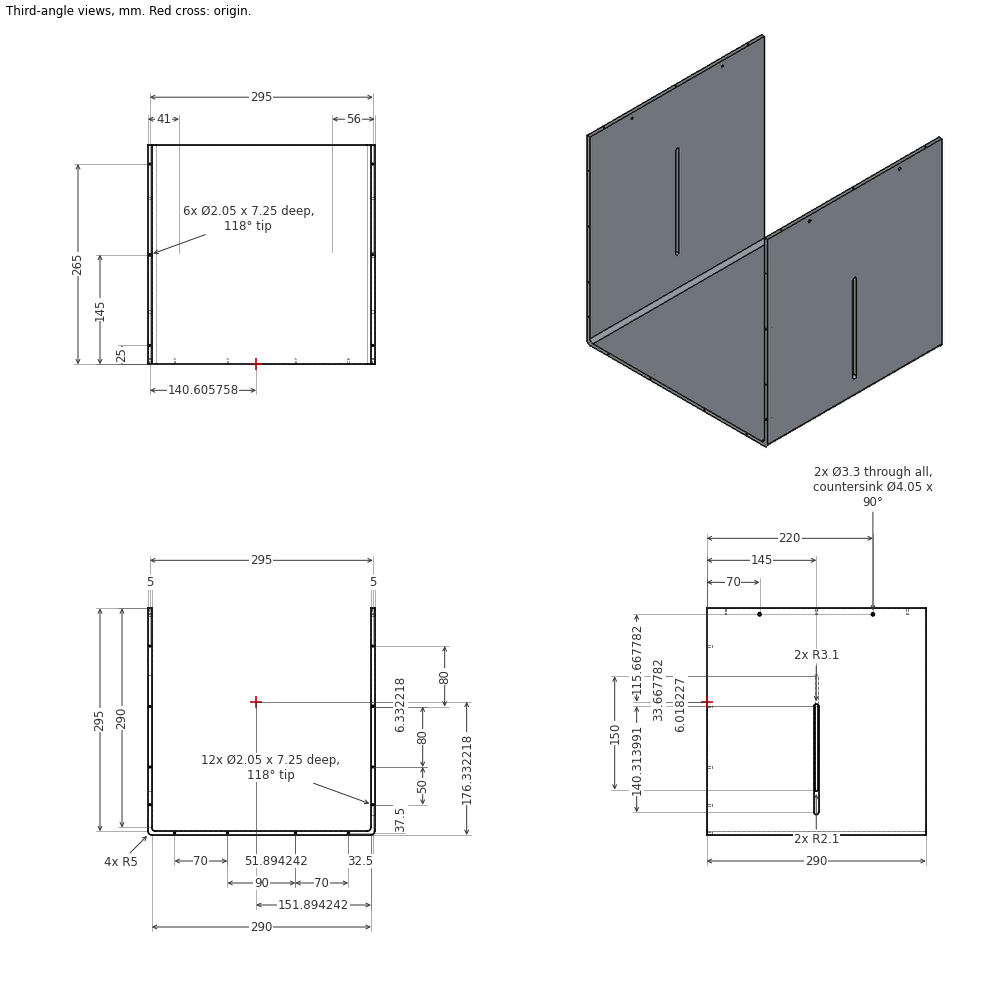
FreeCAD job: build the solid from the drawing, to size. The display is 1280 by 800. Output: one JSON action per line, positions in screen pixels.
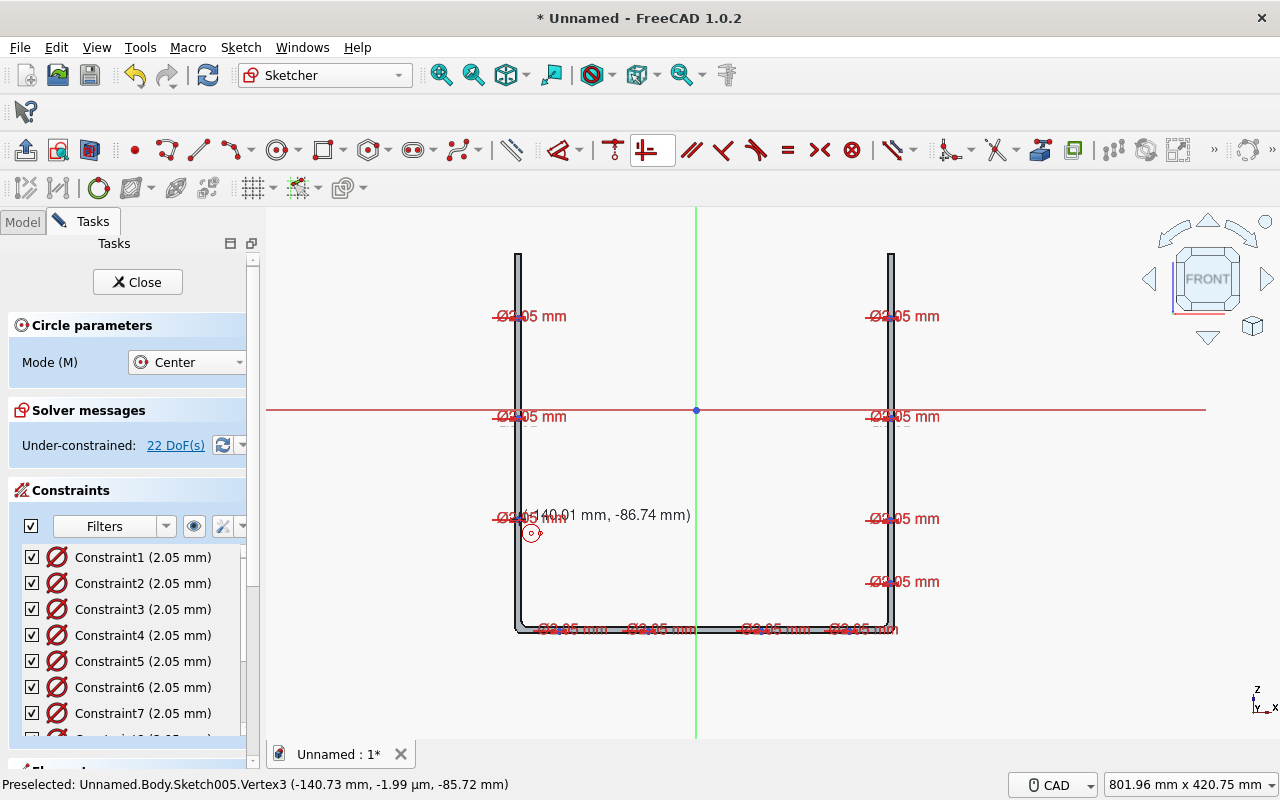
{"action": "scroll", "coordinate": [518, 583], "scroll_direction": "up", "scroll_amount": 15}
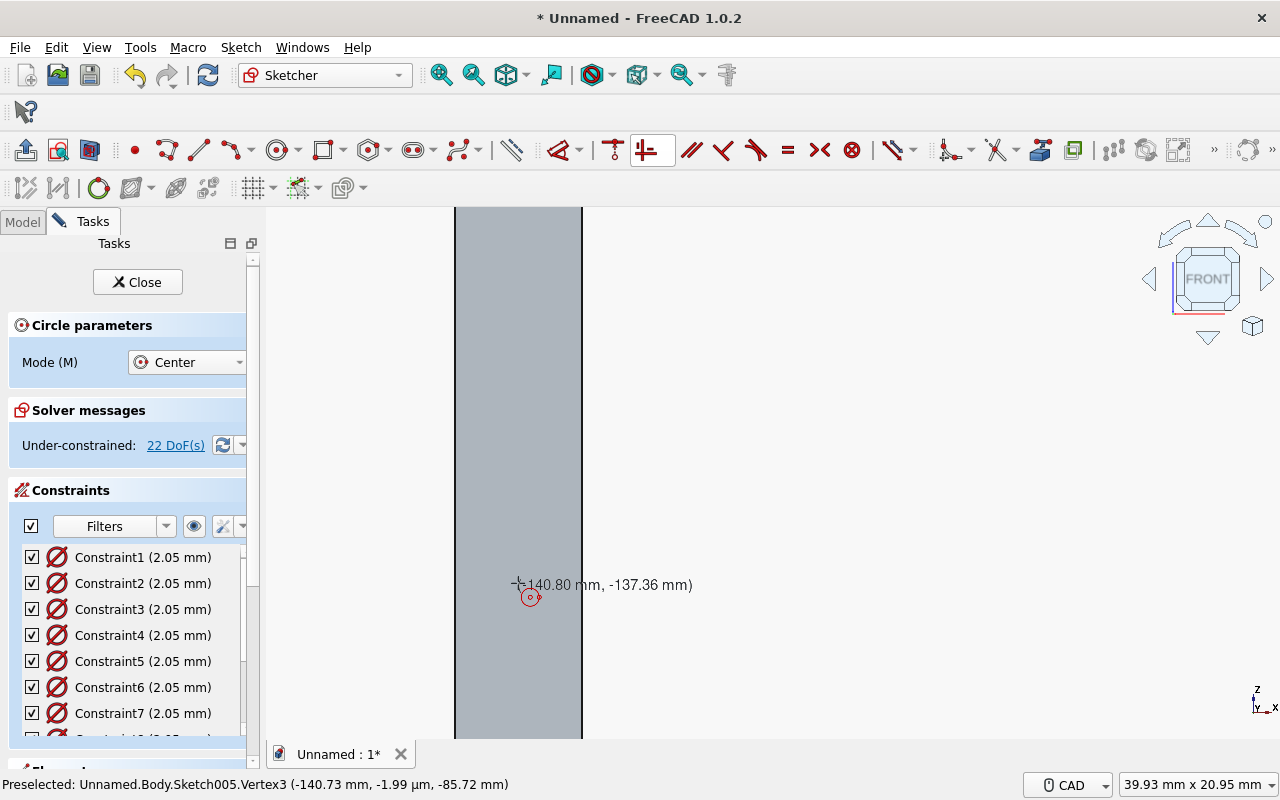
{"action": "scroll", "coordinate": [518, 583], "scroll_direction": "down", "scroll_amount": 15}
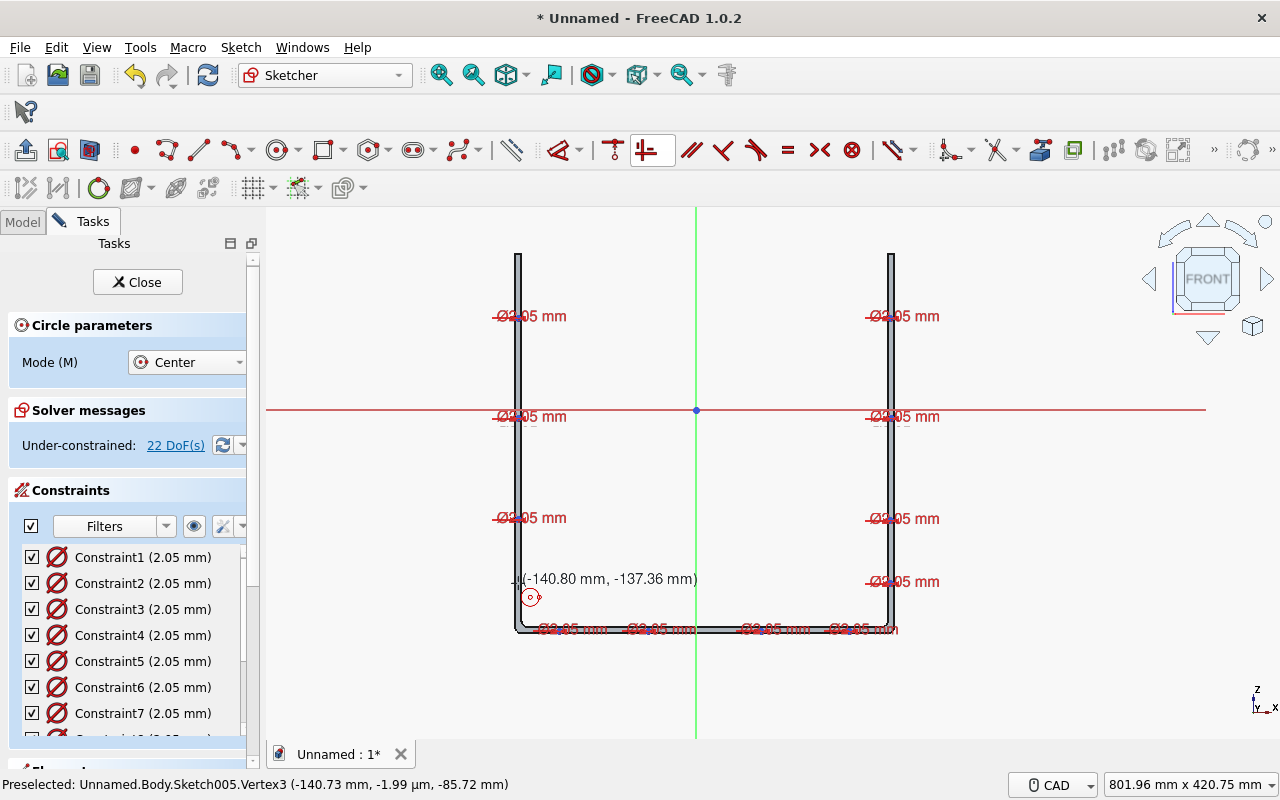
{"action": "left_click", "coordinate": [518, 583]}
{"action": "mouse_move", "coordinate": [519, 582]}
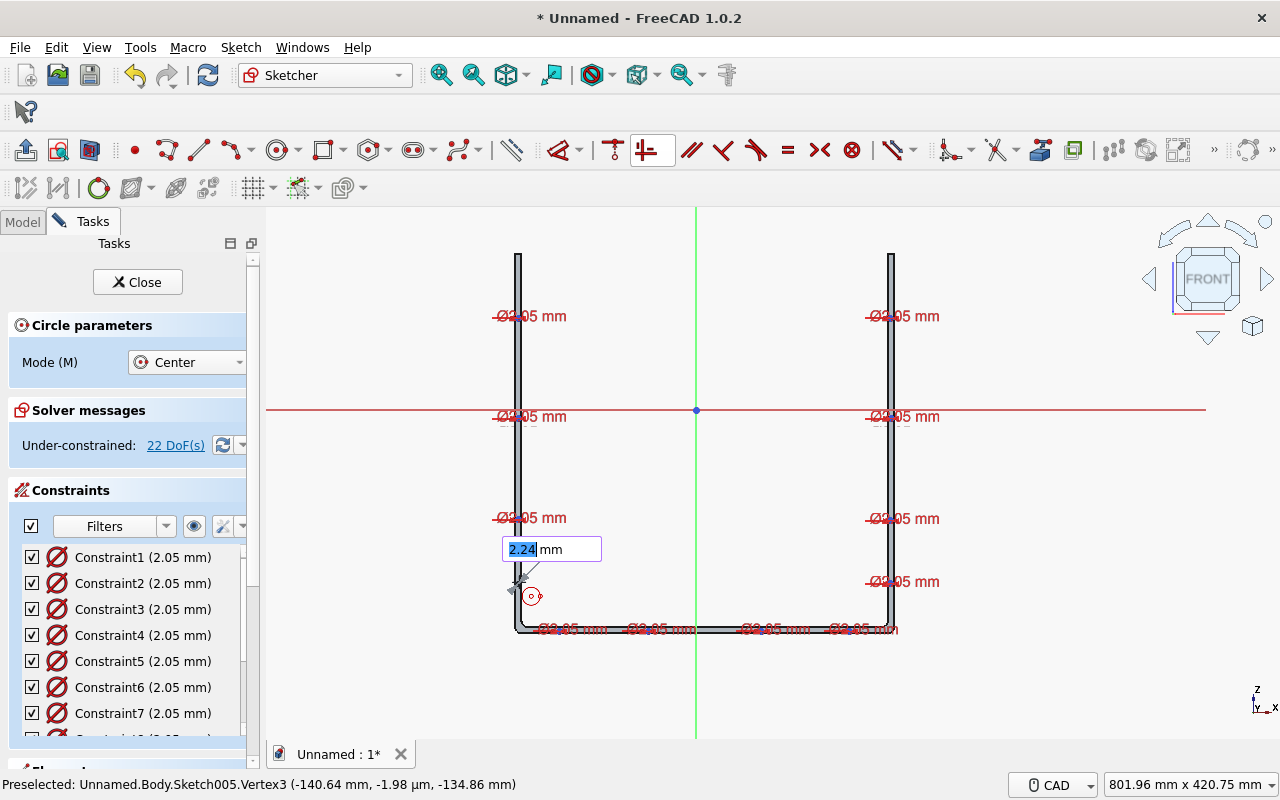
{"action": "type", "text": "2.05"}
{"action": "key", "text": "Return"}
{"action": "key", "text": "Escape"}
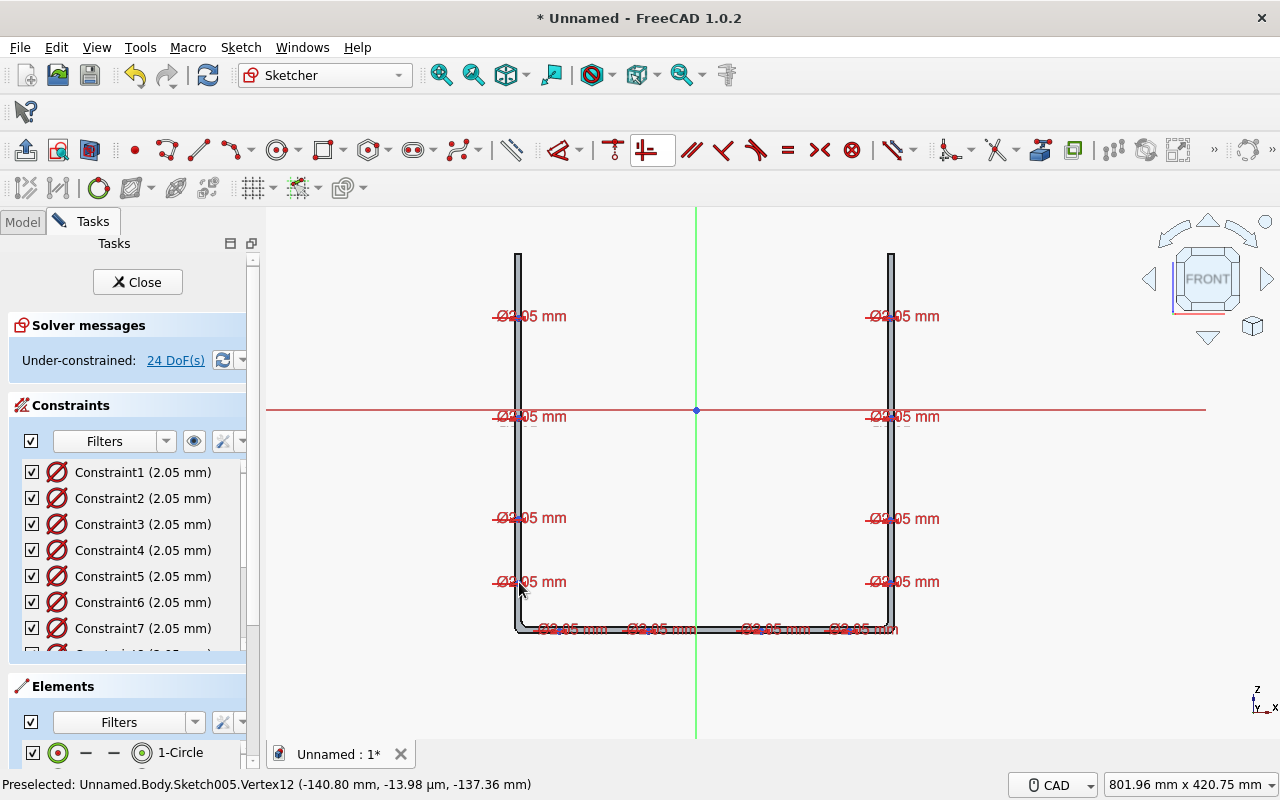
{"action": "left_click", "coordinate": [891, 584]}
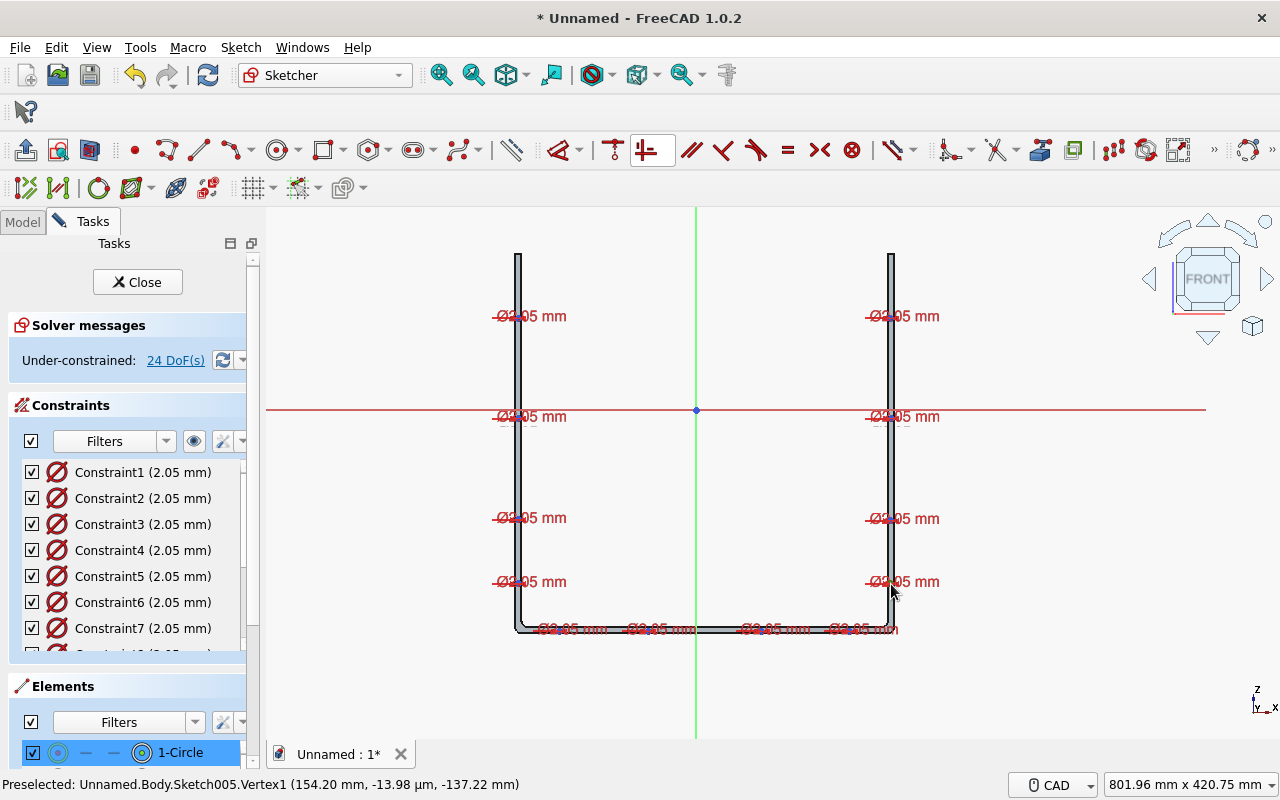
{"action": "left_click", "coordinate": [891, 521]}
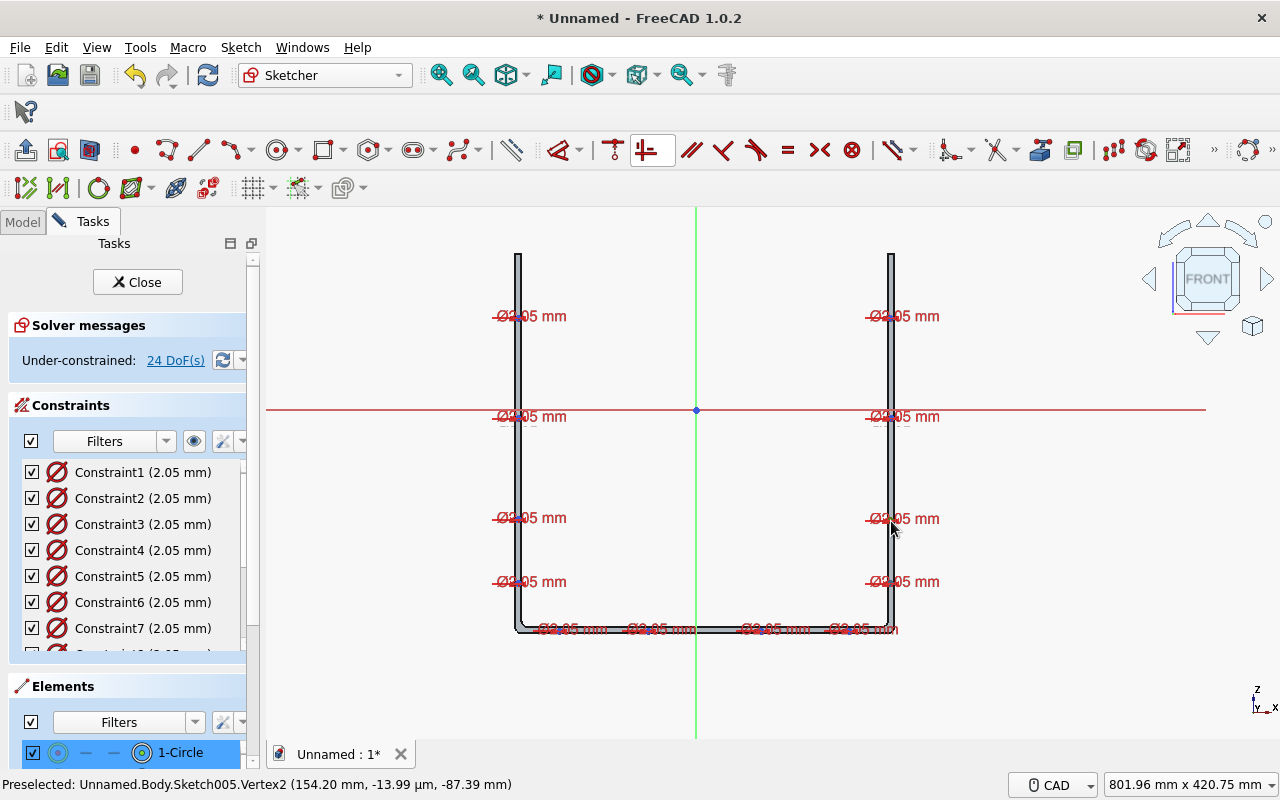
{"action": "left_click", "coordinate": [670, 150]}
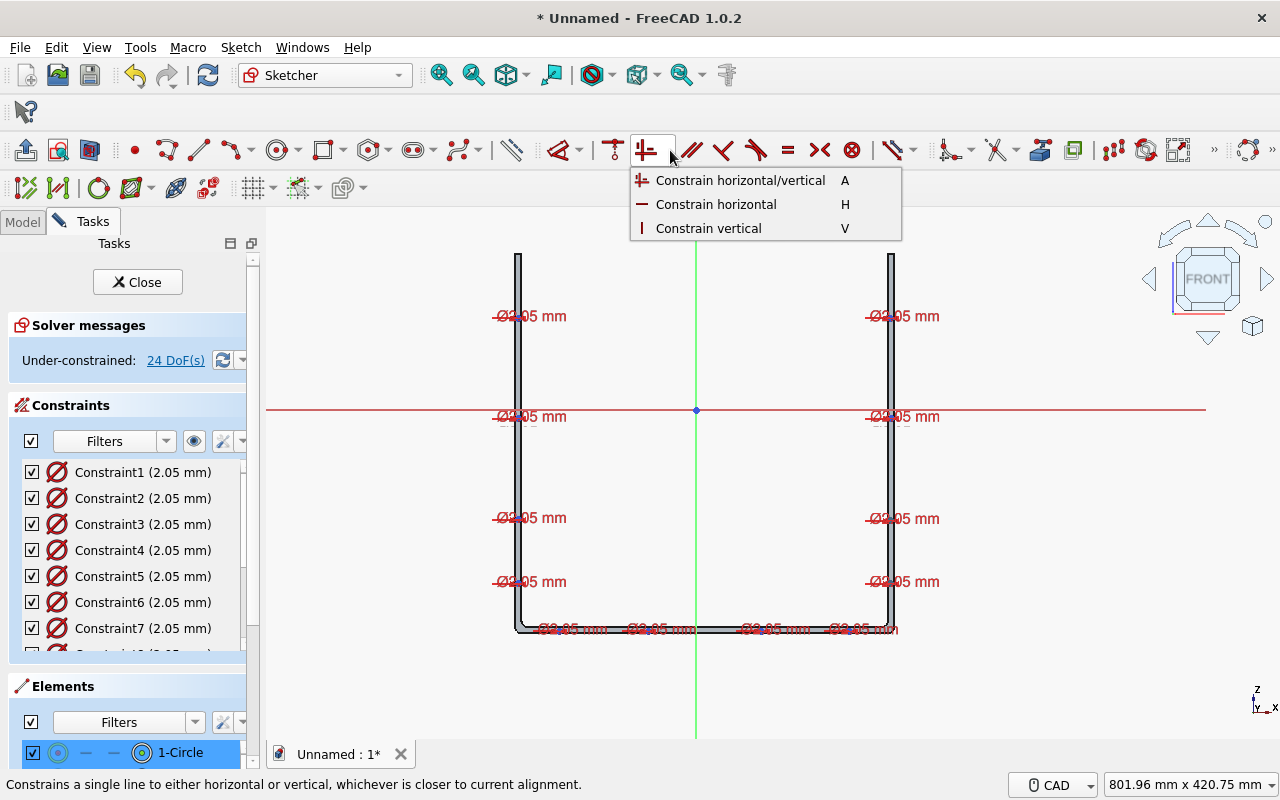
{"action": "left_click", "coordinate": [766, 228]}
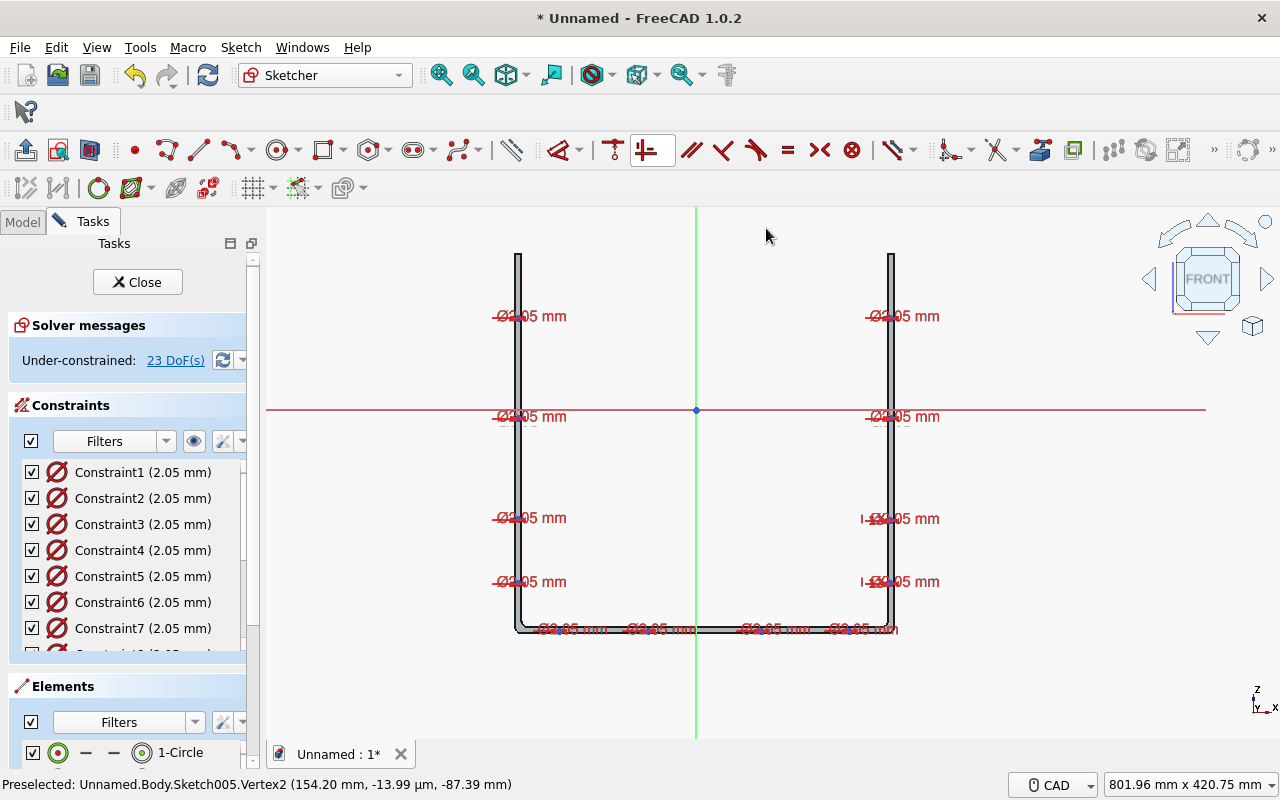
{"action": "left_click", "coordinate": [891, 521]}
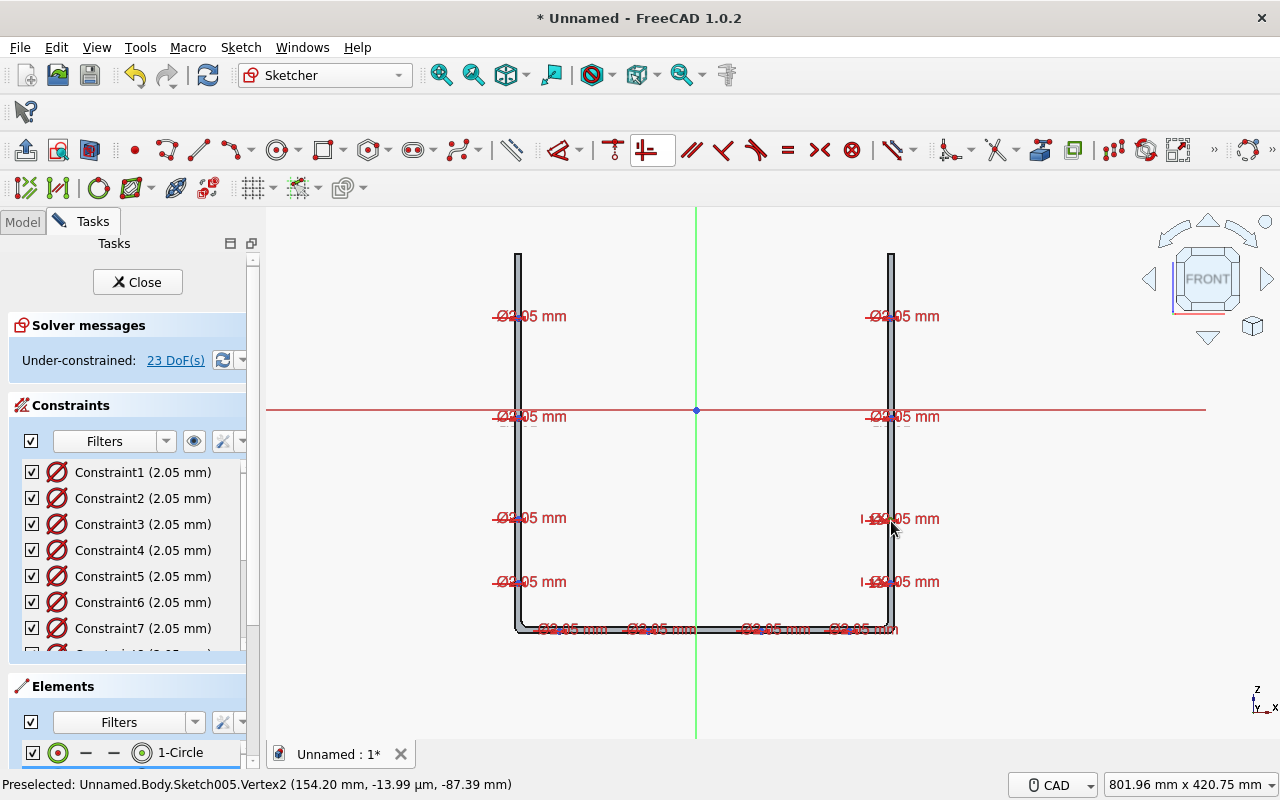
{"action": "left_click", "coordinate": [891, 419]}